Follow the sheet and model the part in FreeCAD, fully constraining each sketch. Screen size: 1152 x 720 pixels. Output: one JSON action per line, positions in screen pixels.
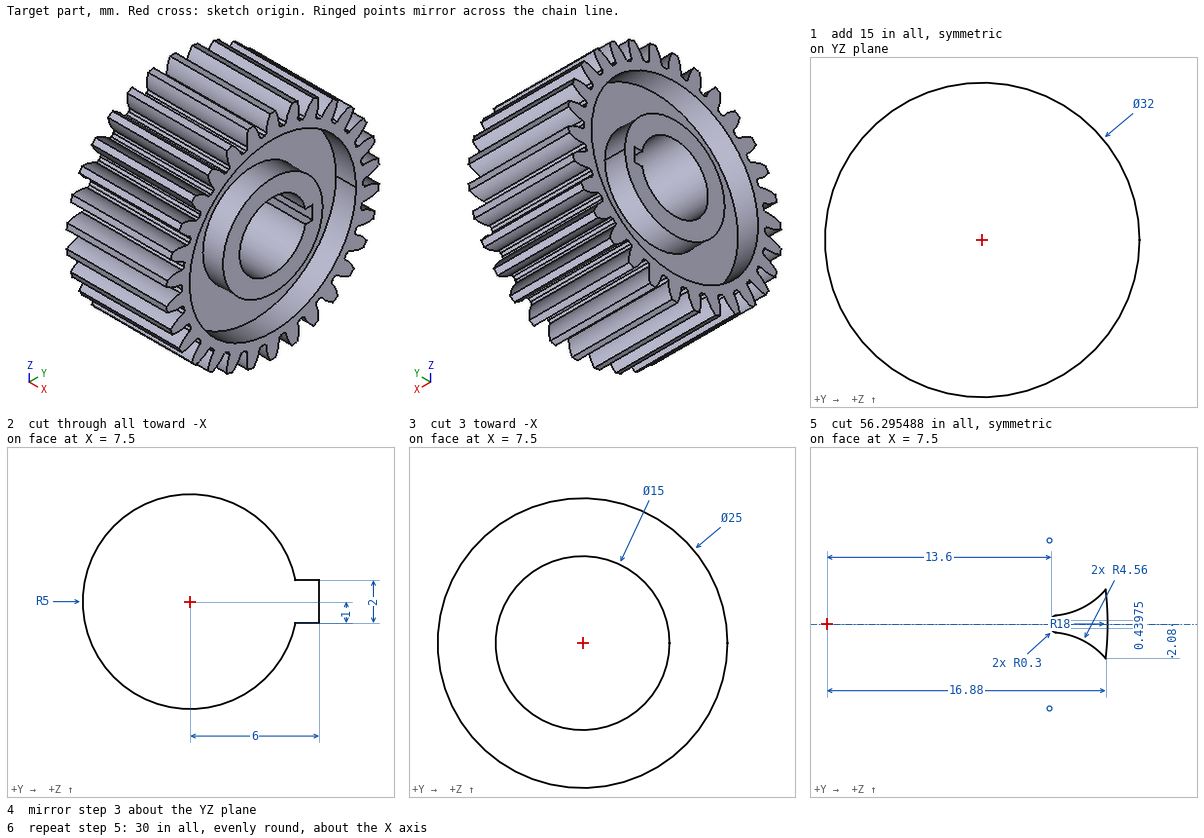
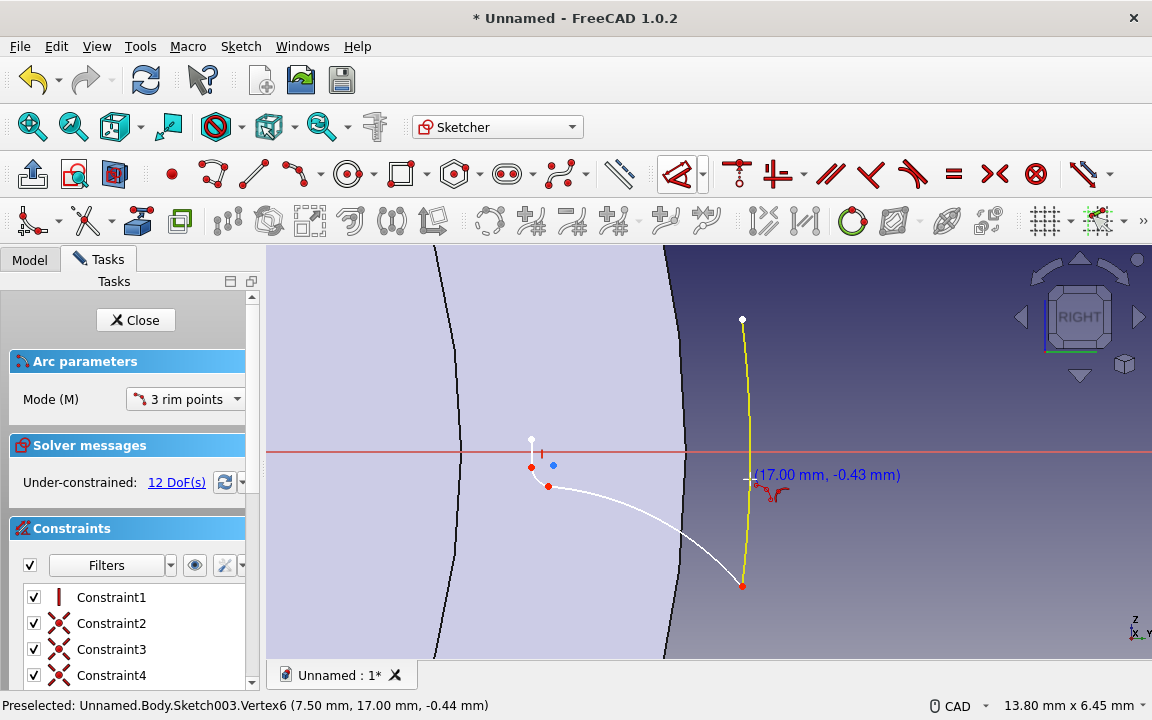
{"action": "left_click", "coordinate": [742, 320]}
{"action": "left_click", "coordinate": [549, 419]}
{"action": "left_click", "coordinate": [656, 388]}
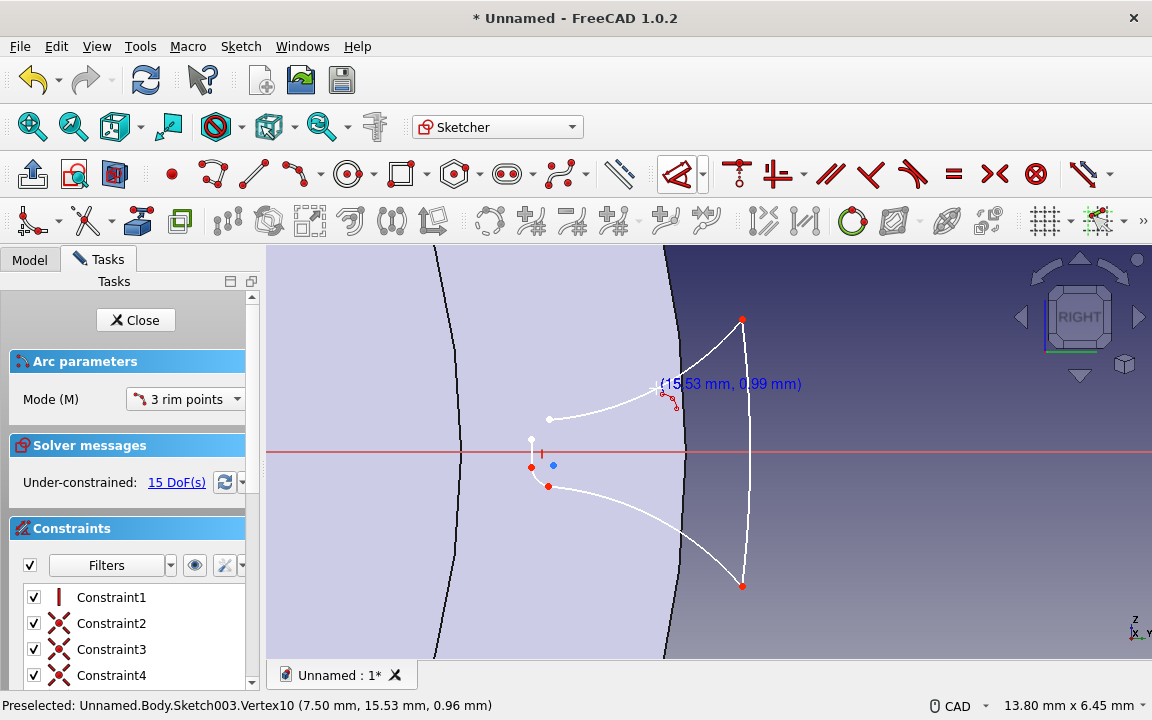
{"action": "left_click", "coordinate": [549, 420]}
{"action": "left_click", "coordinate": [532, 440]}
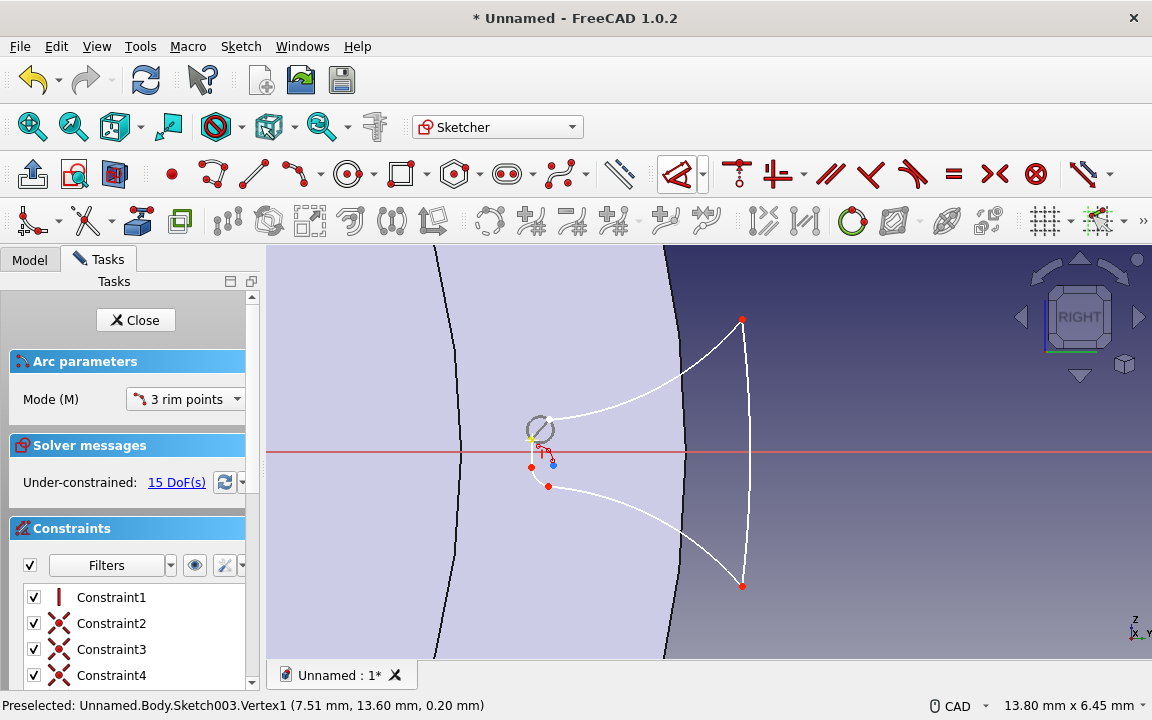
{"action": "scroll", "coordinate": [537, 425], "scroll_direction": "up", "scroll_amount": 6}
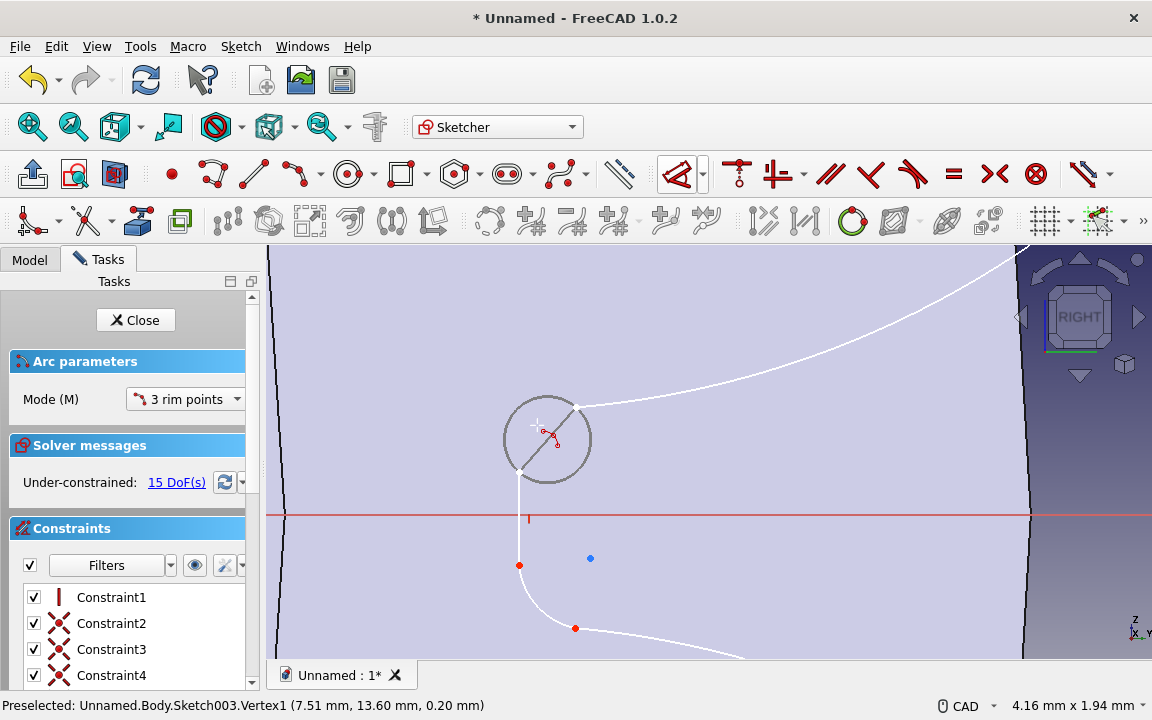
{"action": "left_click", "coordinate": [536, 425]}
{"action": "key", "text": "Escape"}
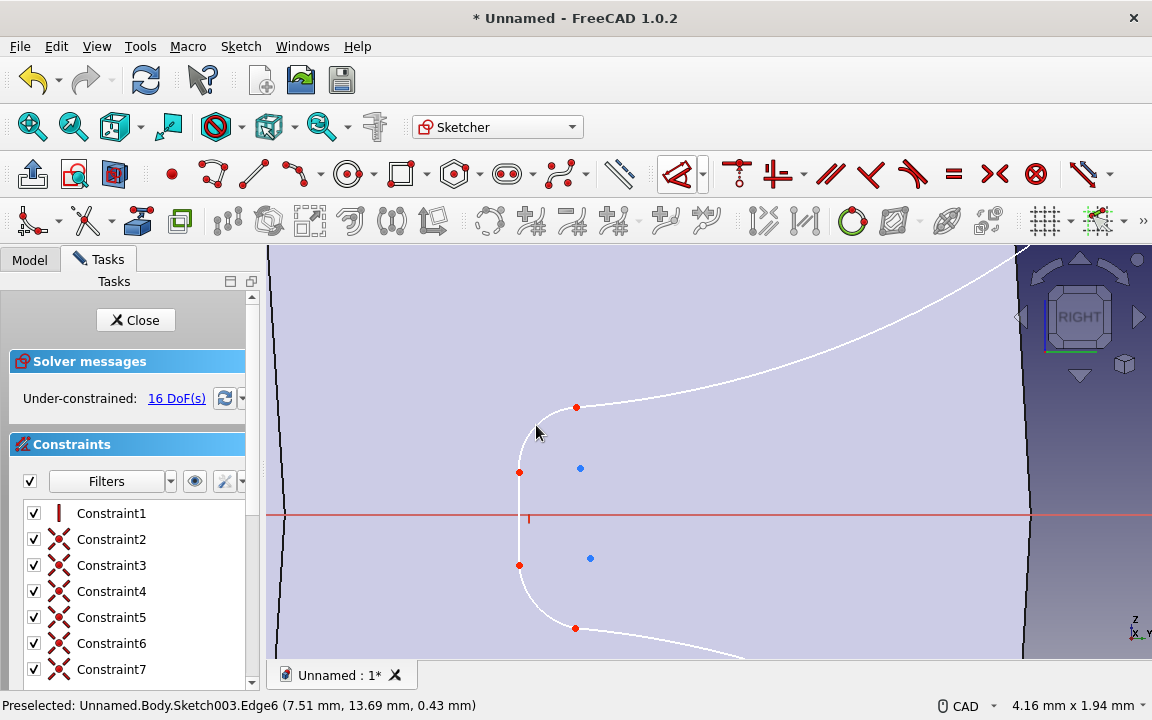
{"action": "left_click", "coordinate": [519, 500]}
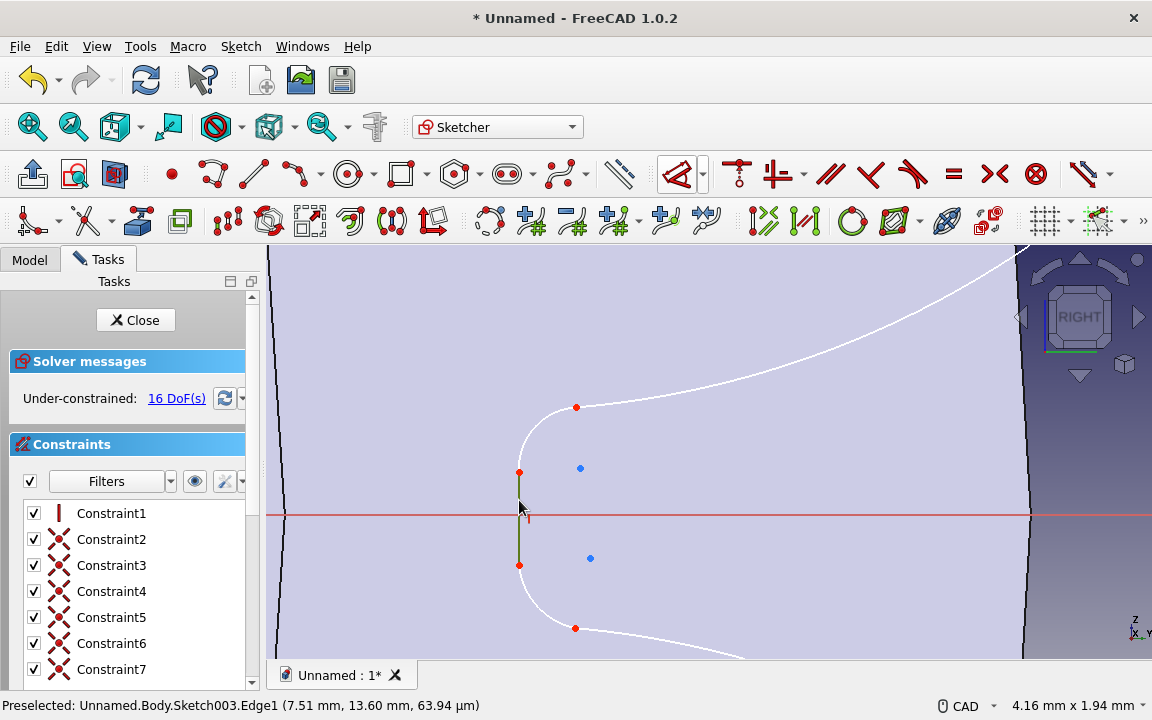
{"action": "left_click", "coordinate": [527, 591]}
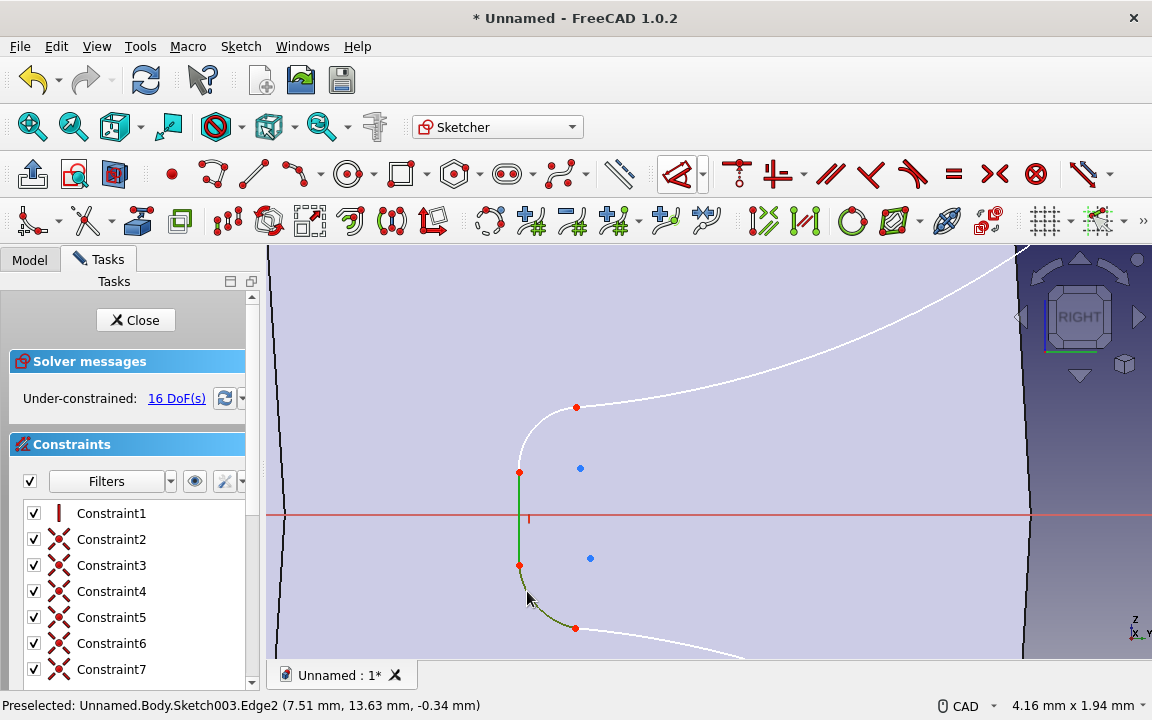
{"action": "key", "text": "t"}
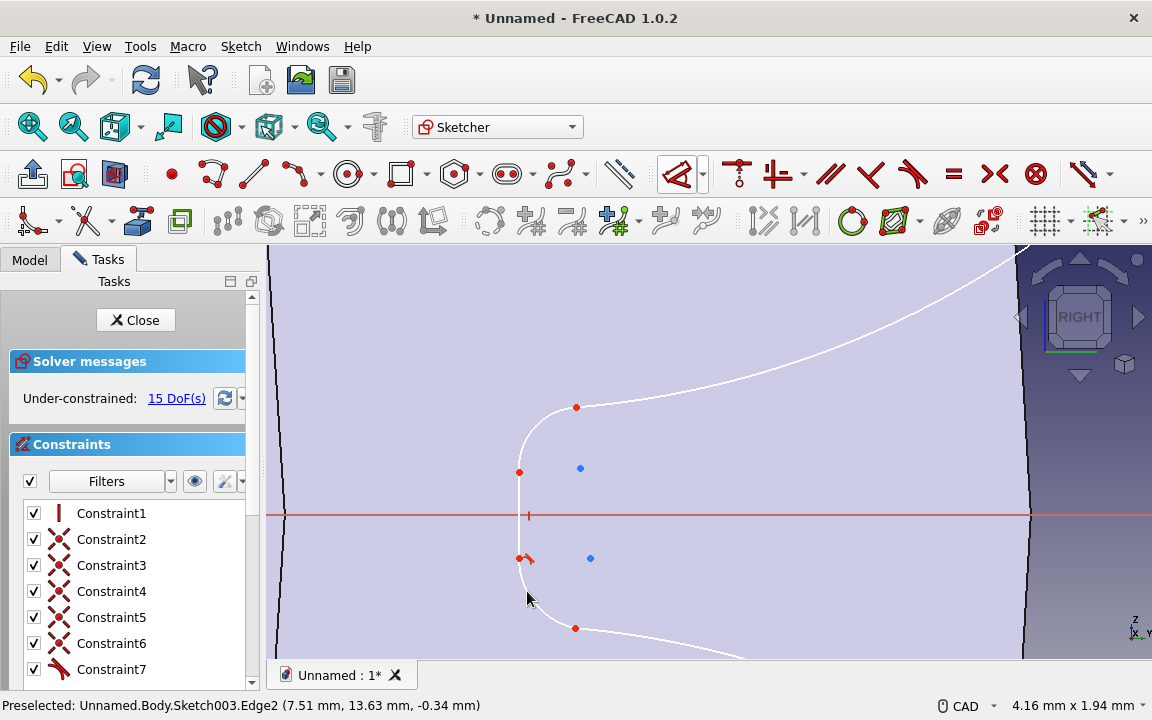
{"action": "left_click", "coordinate": [519, 498]}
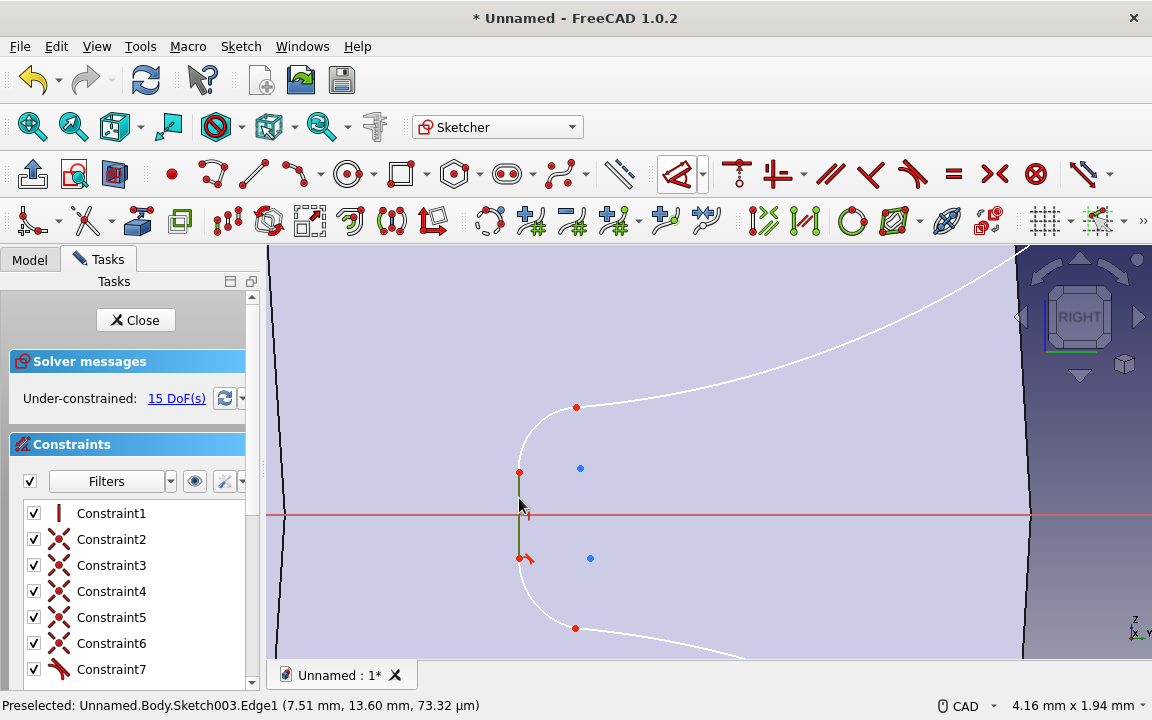
{"action": "left_click", "coordinate": [549, 416]}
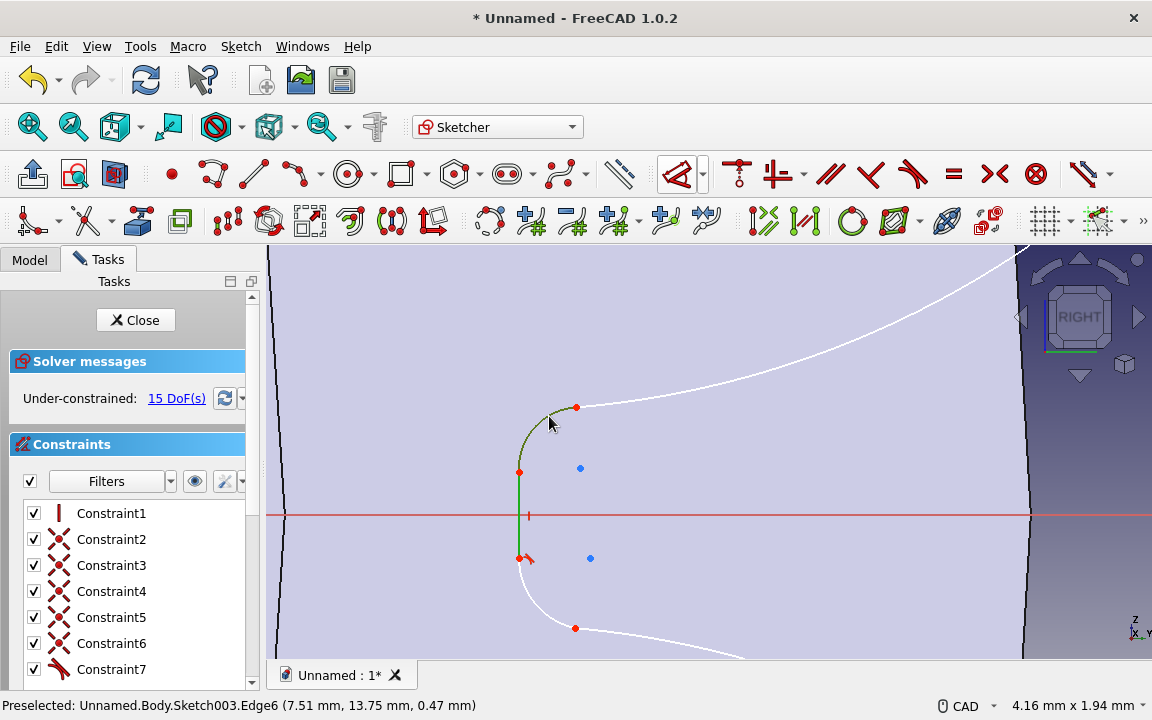
{"action": "left_click", "coordinate": [913, 174]}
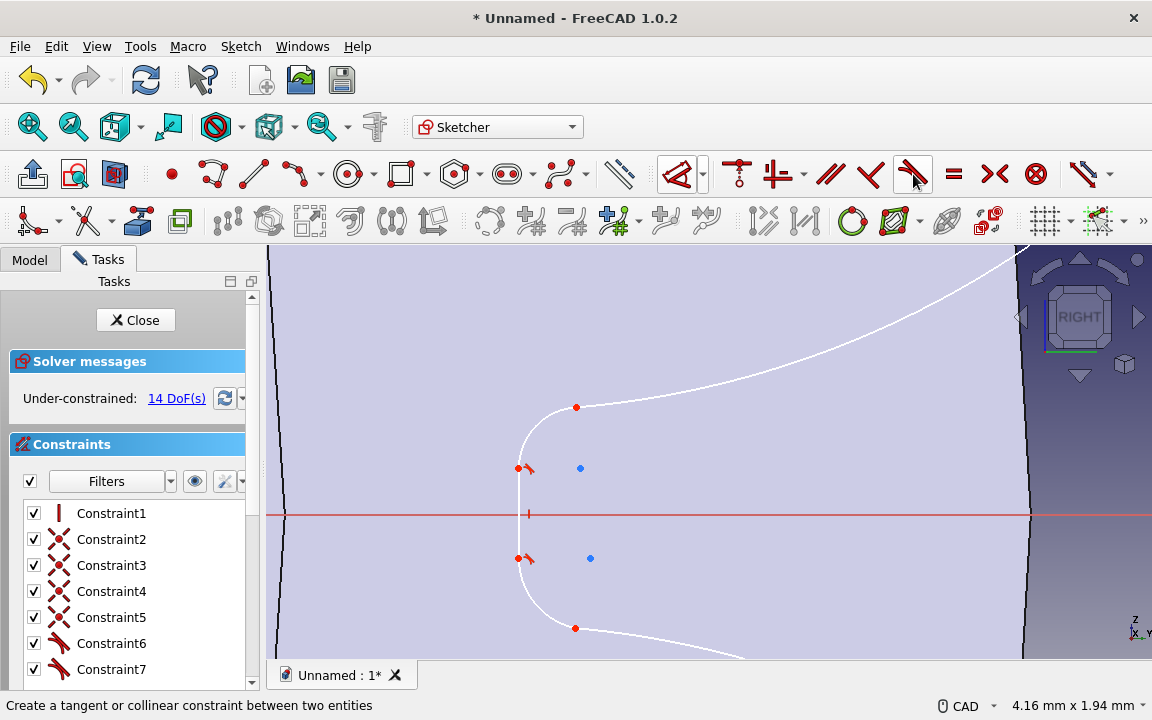
{"action": "left_click", "coordinate": [525, 587]}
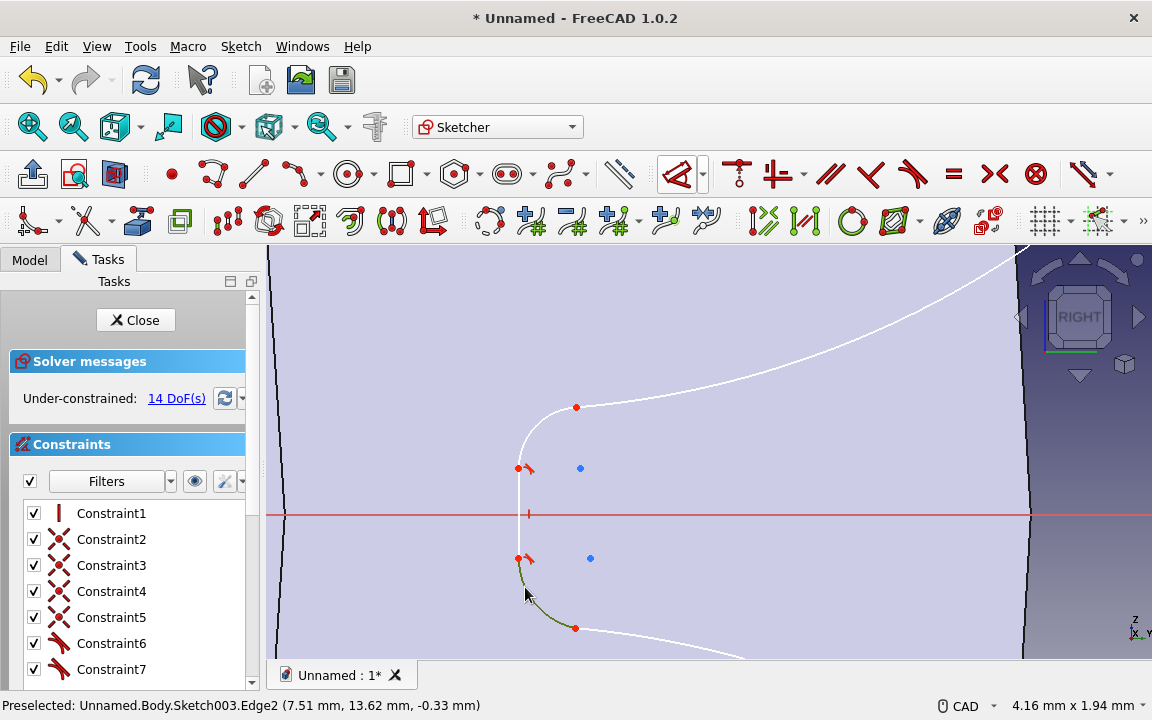
{"action": "scroll", "coordinate": [537, 425], "scroll_direction": "down", "scroll_amount": 6}